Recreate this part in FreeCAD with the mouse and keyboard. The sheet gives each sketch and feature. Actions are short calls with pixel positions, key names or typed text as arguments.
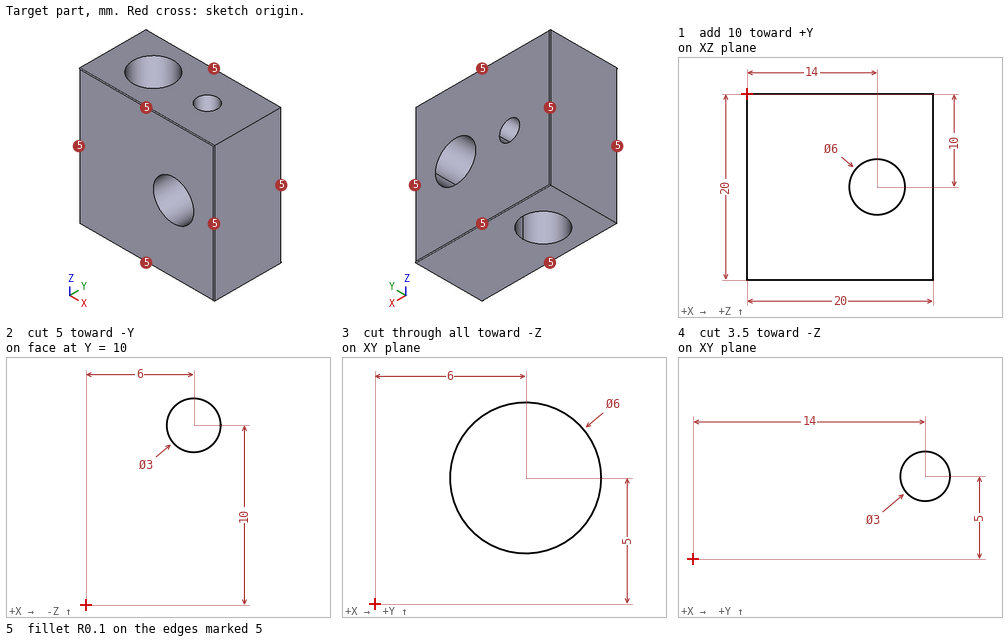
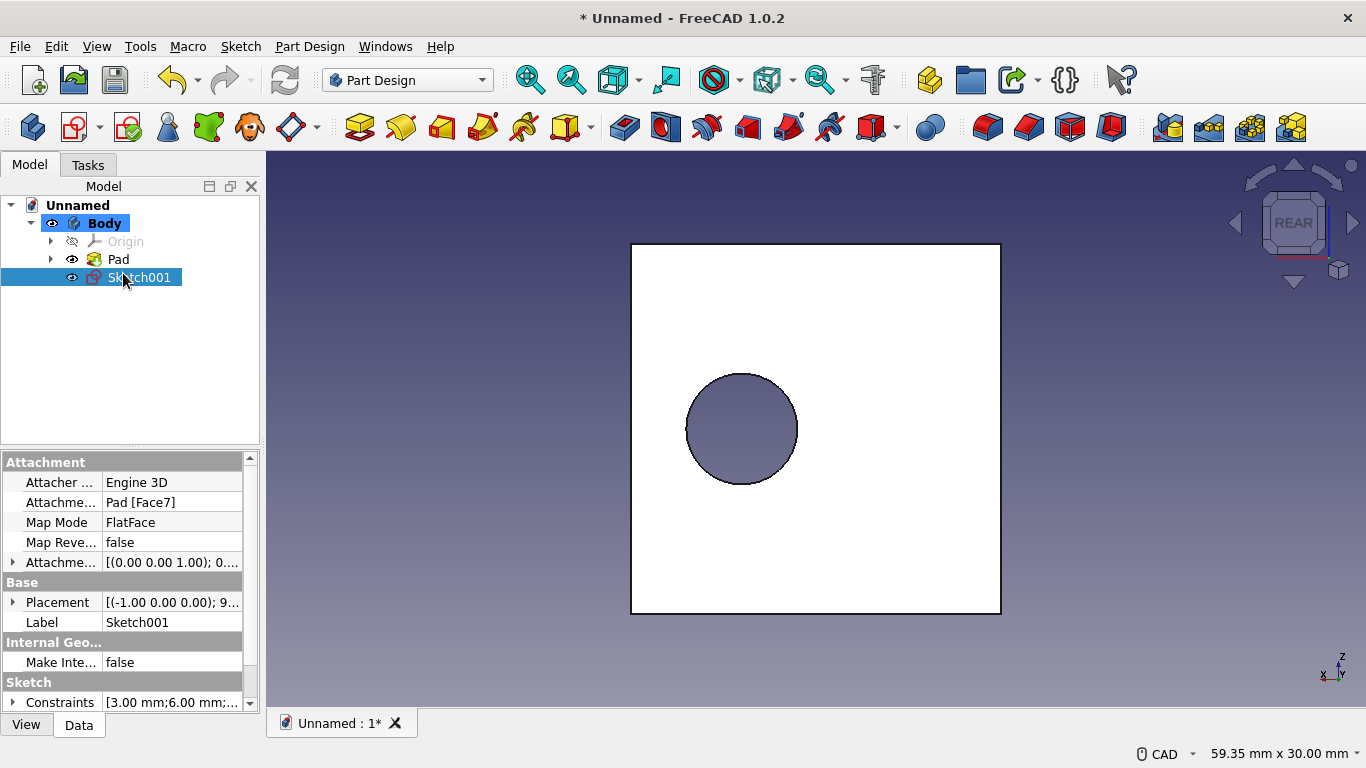
click(625, 128)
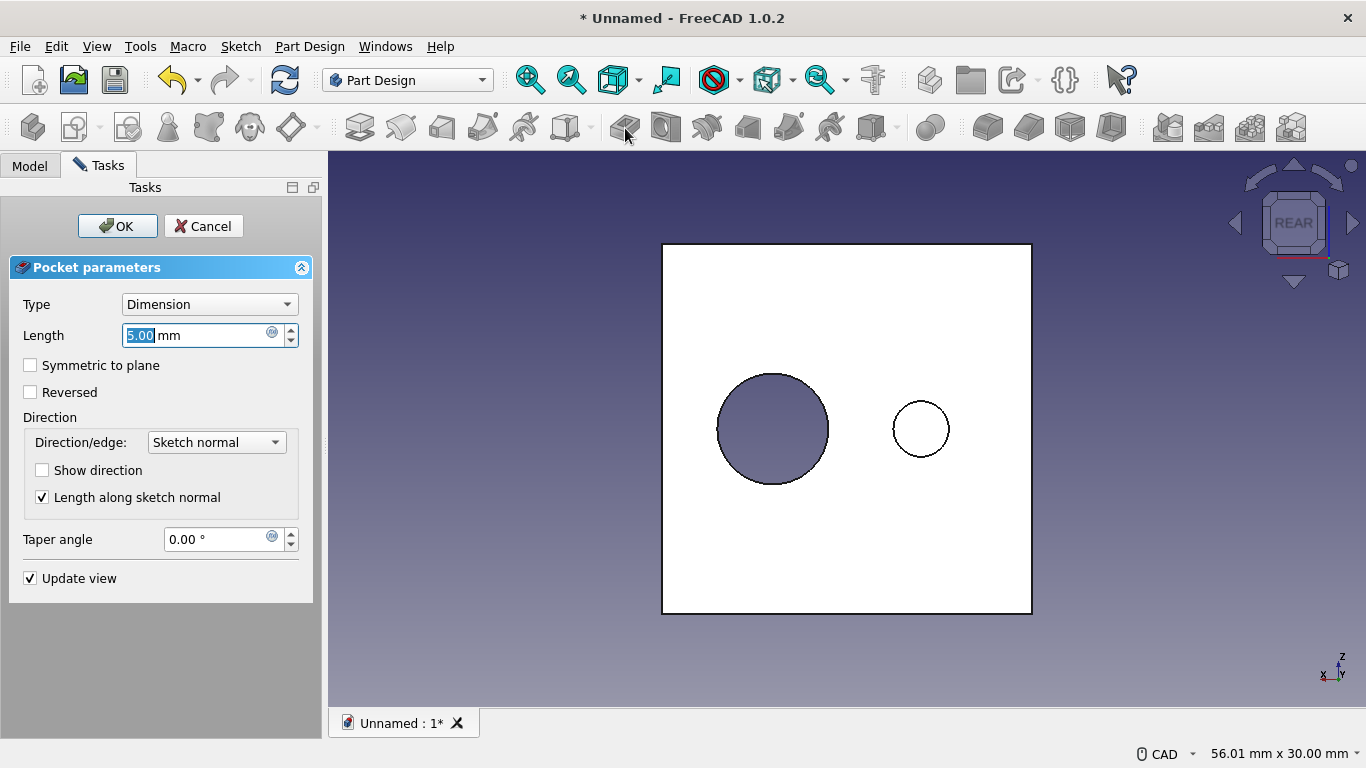
text(5)
key(Tab)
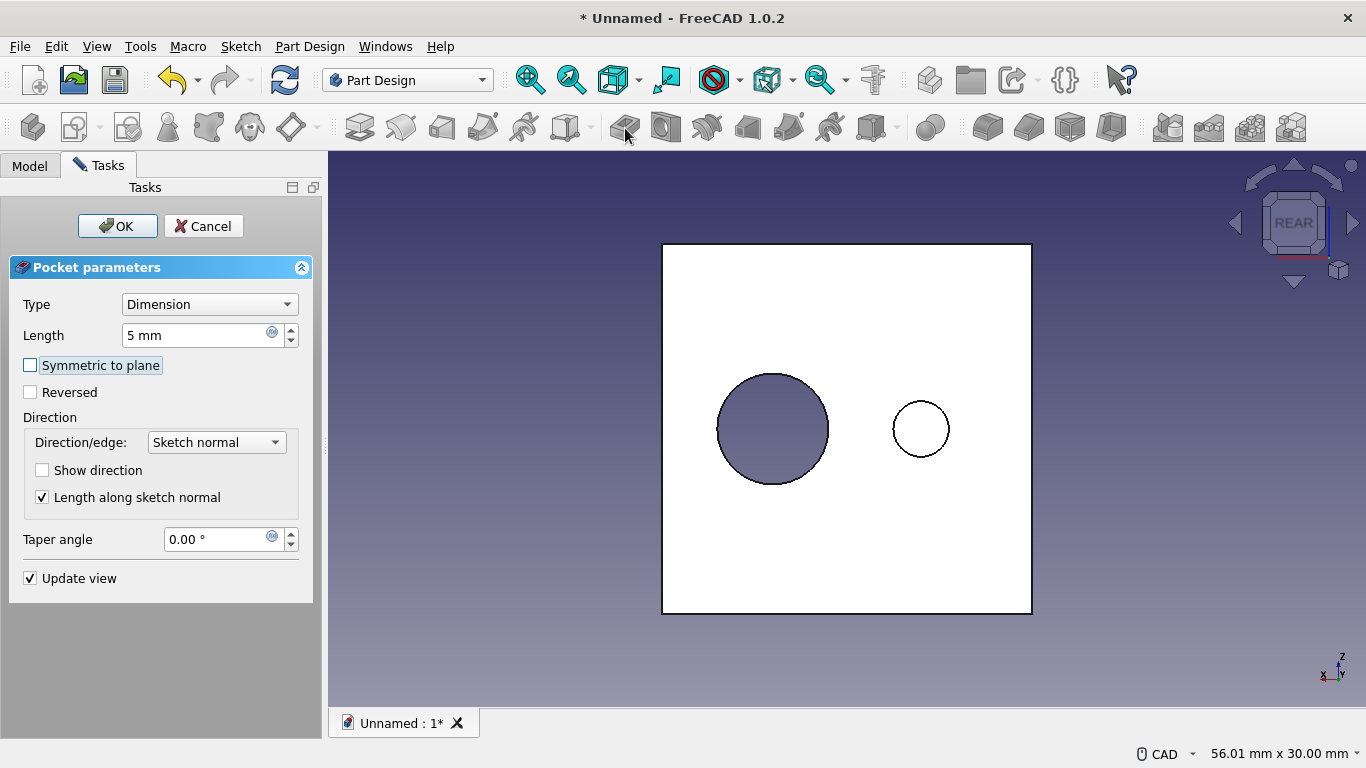
click(118, 226)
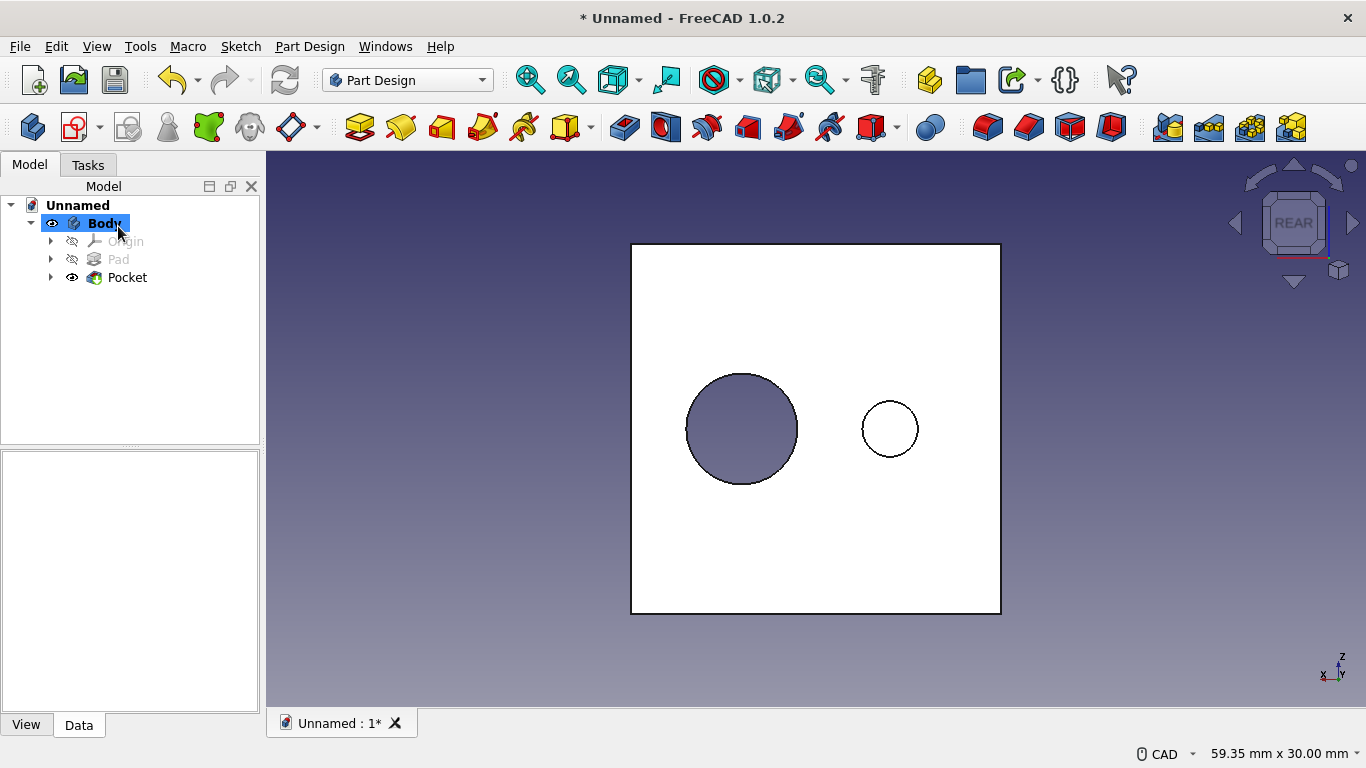
click(74, 128)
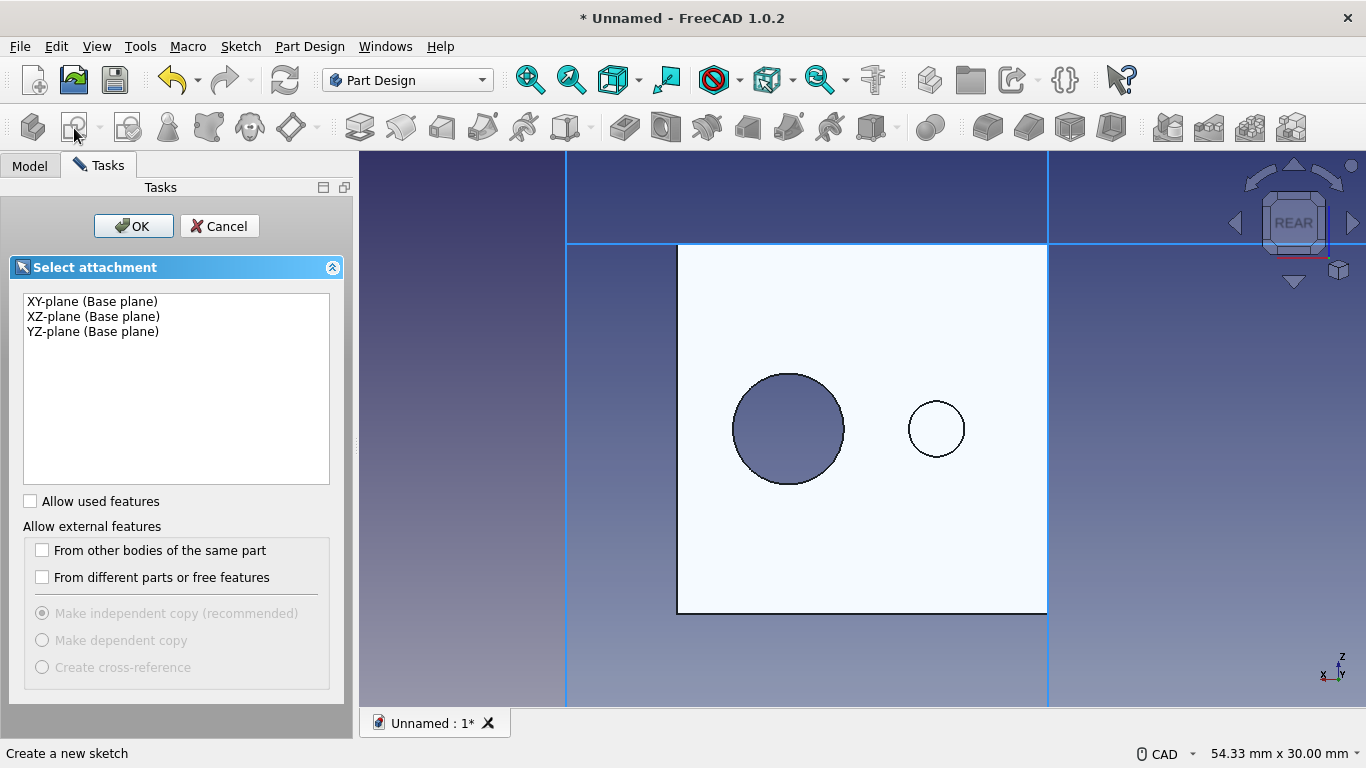
click(84, 302)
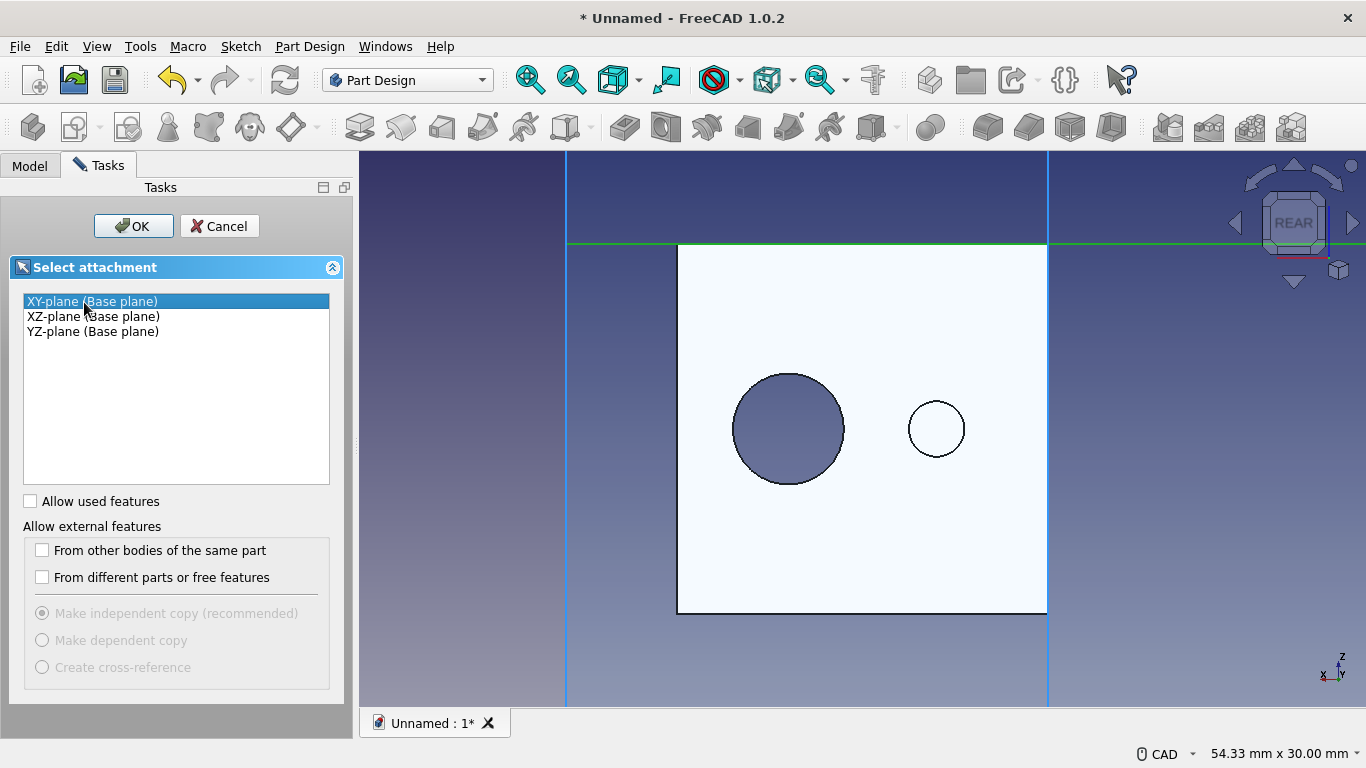
click(134, 226)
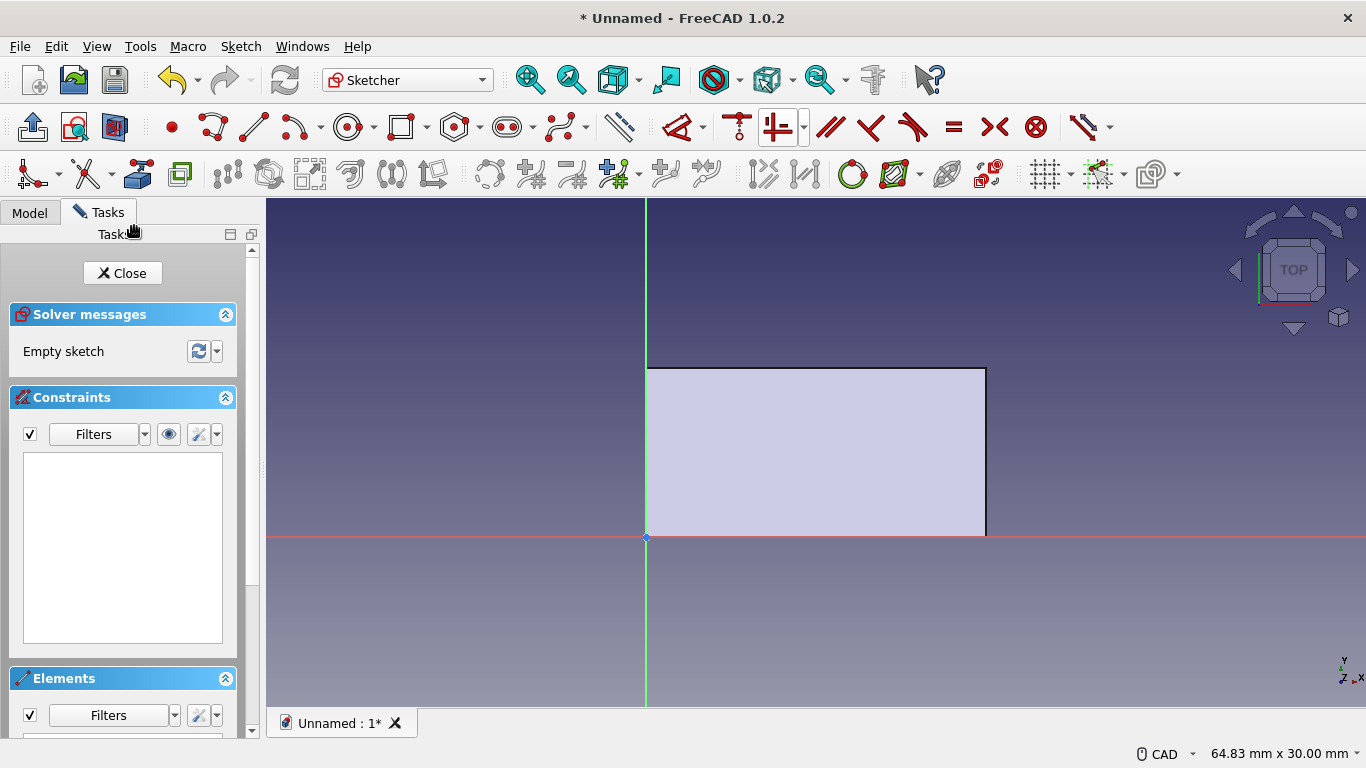
scroll(702, 483, up, 4)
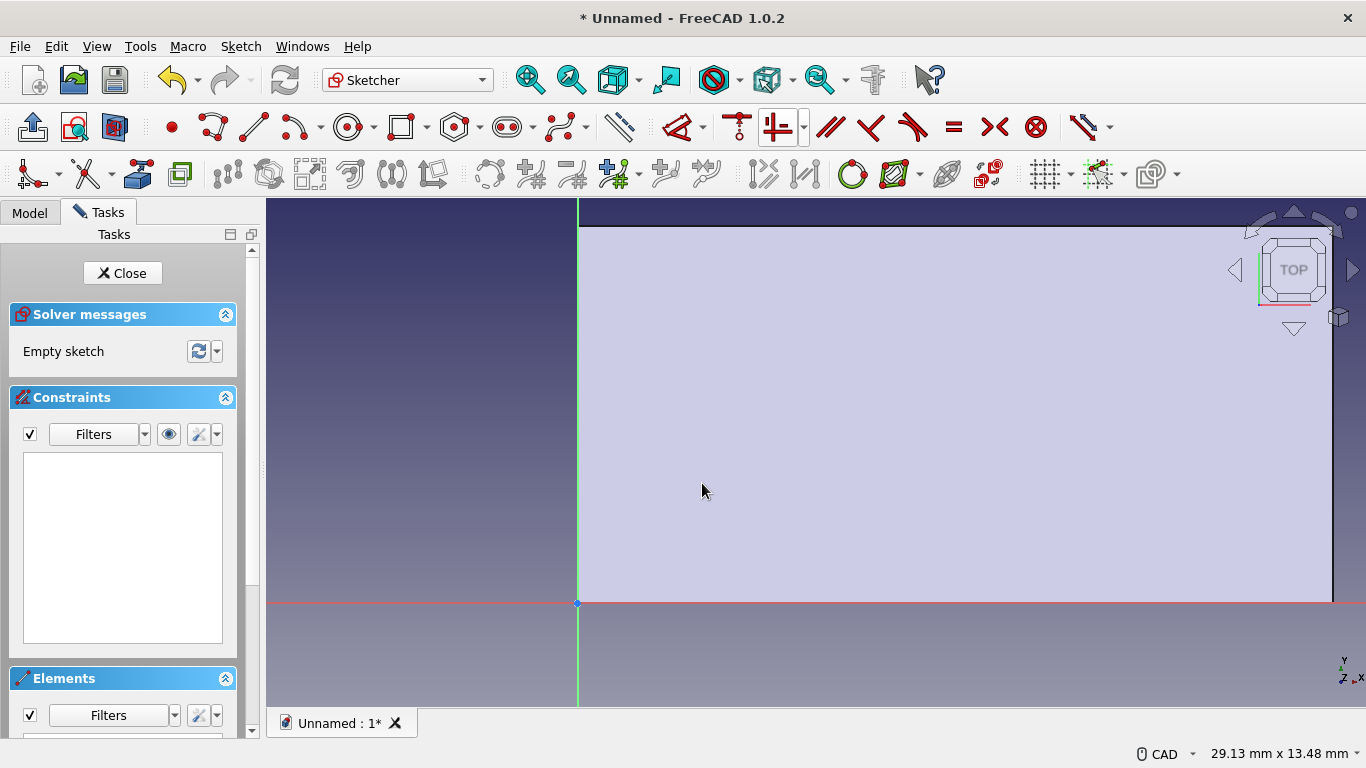
click(348, 128)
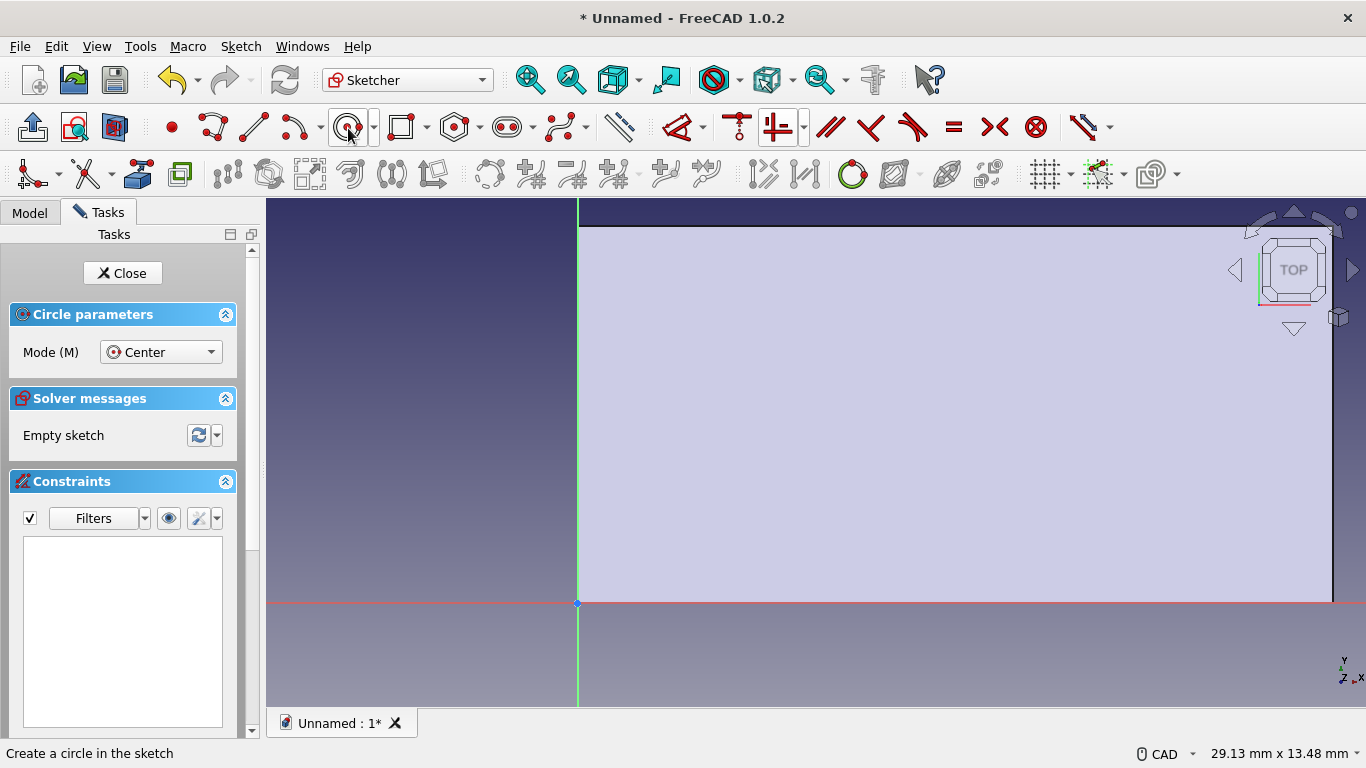
click(804, 414)
click(884, 334)
key(Escape)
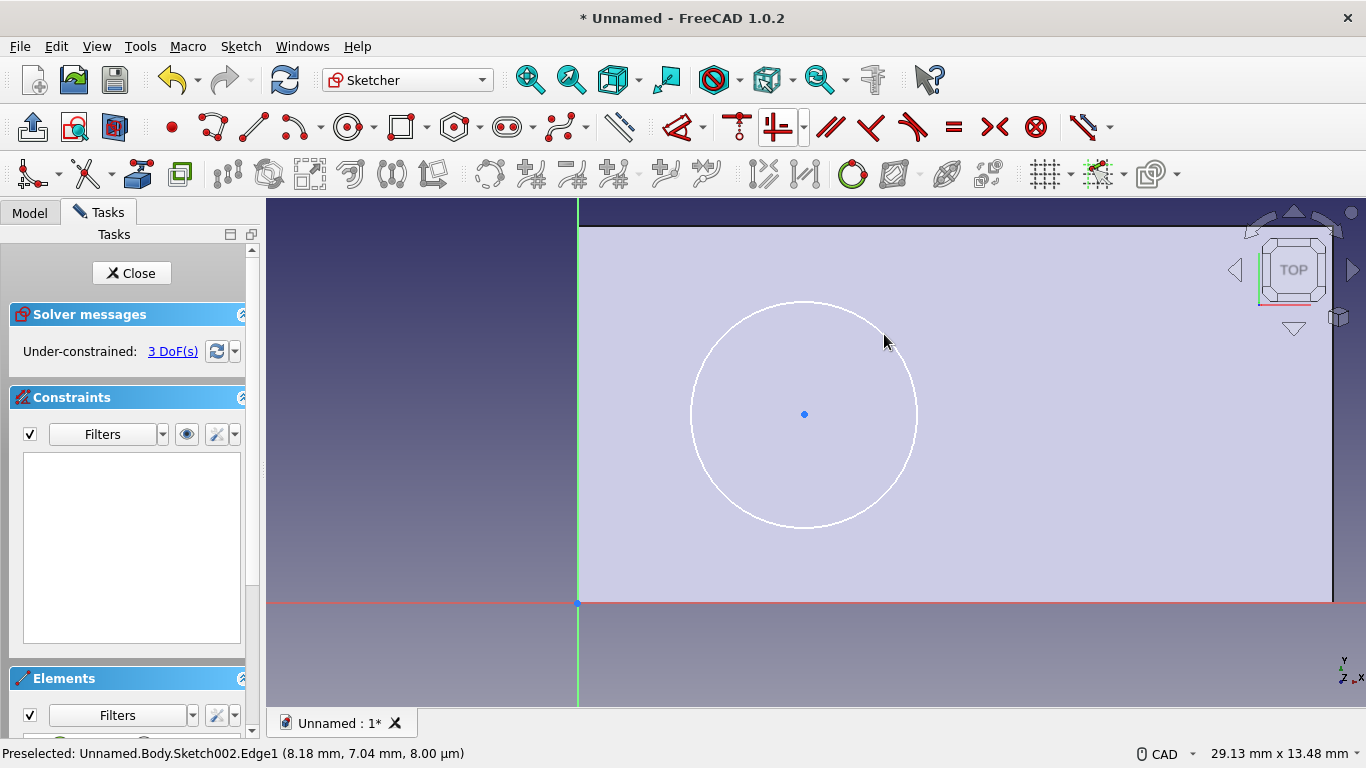
click(676, 128)